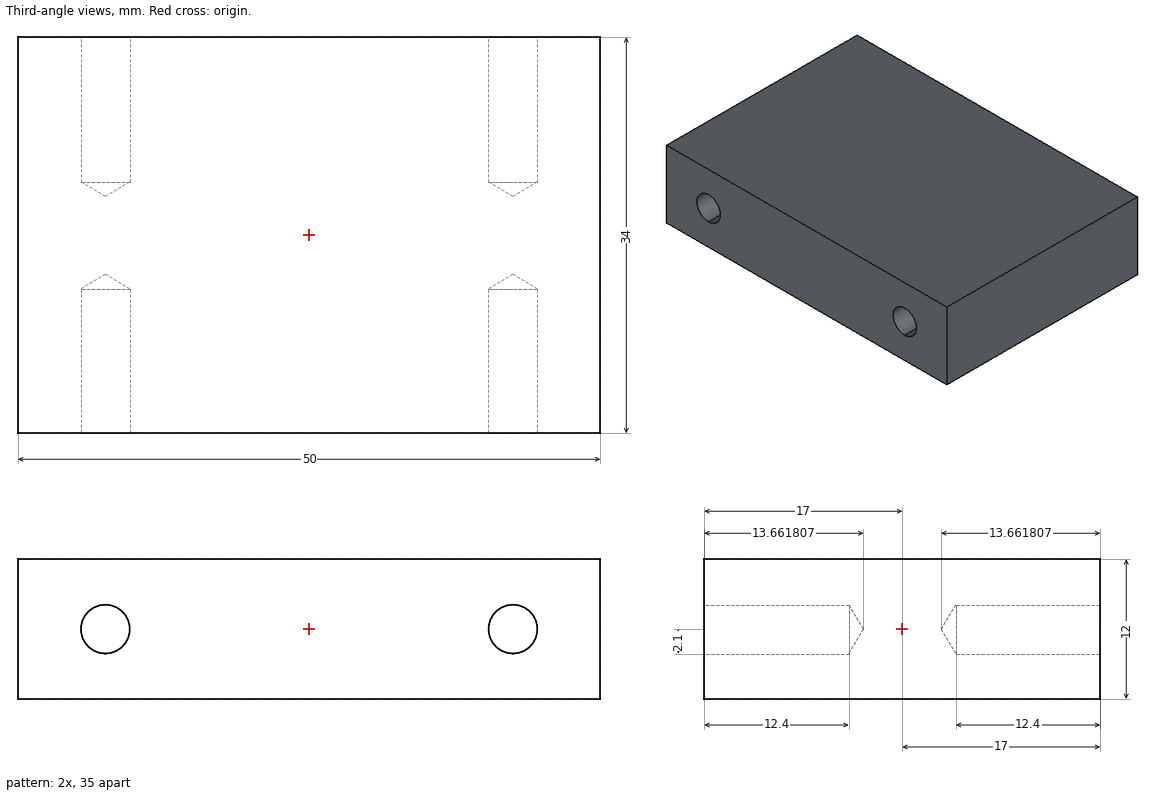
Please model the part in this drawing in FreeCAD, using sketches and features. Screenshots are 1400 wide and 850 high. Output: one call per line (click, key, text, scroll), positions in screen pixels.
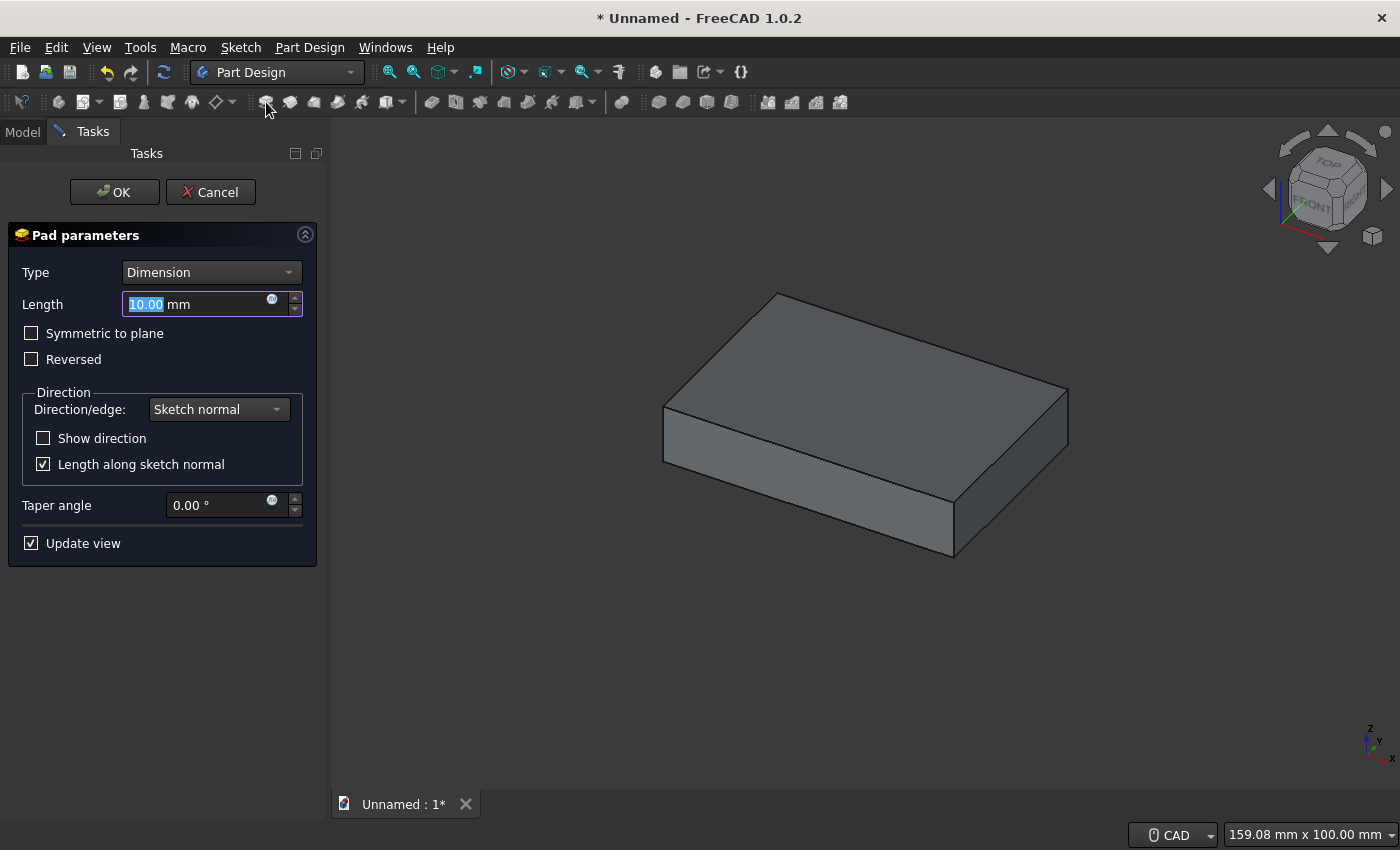
text(12)
key(Tab)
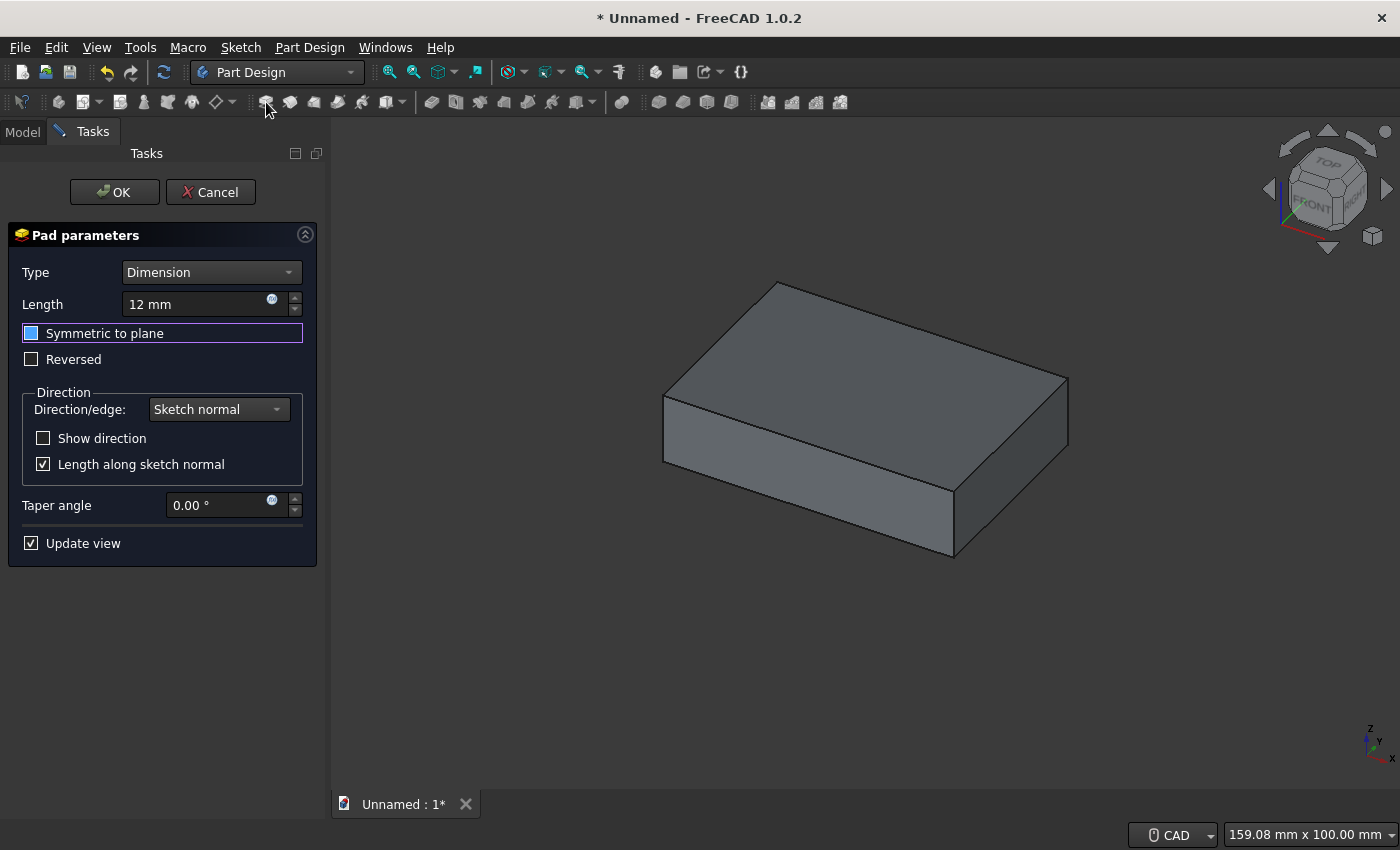
click(30, 333)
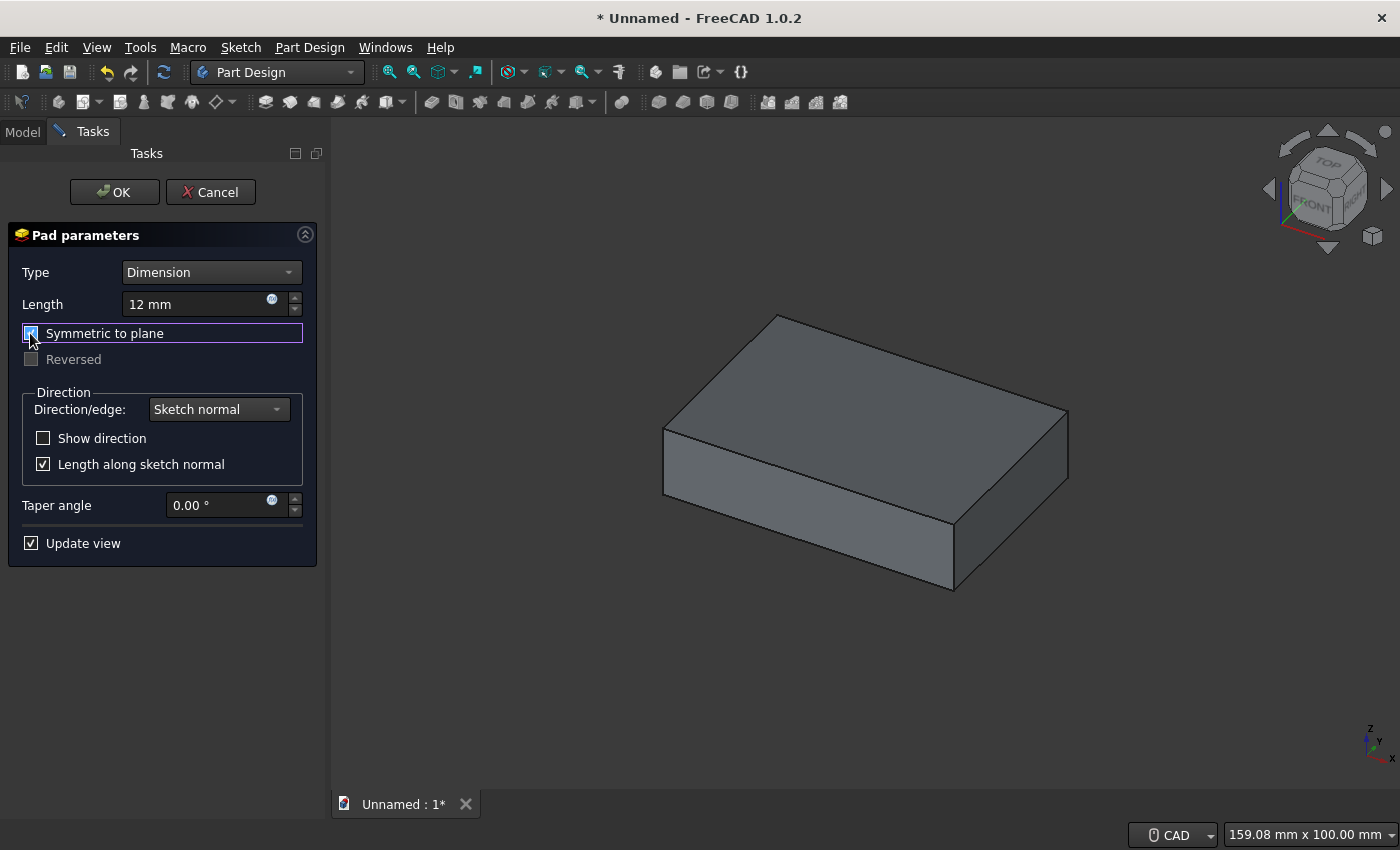
click(115, 192)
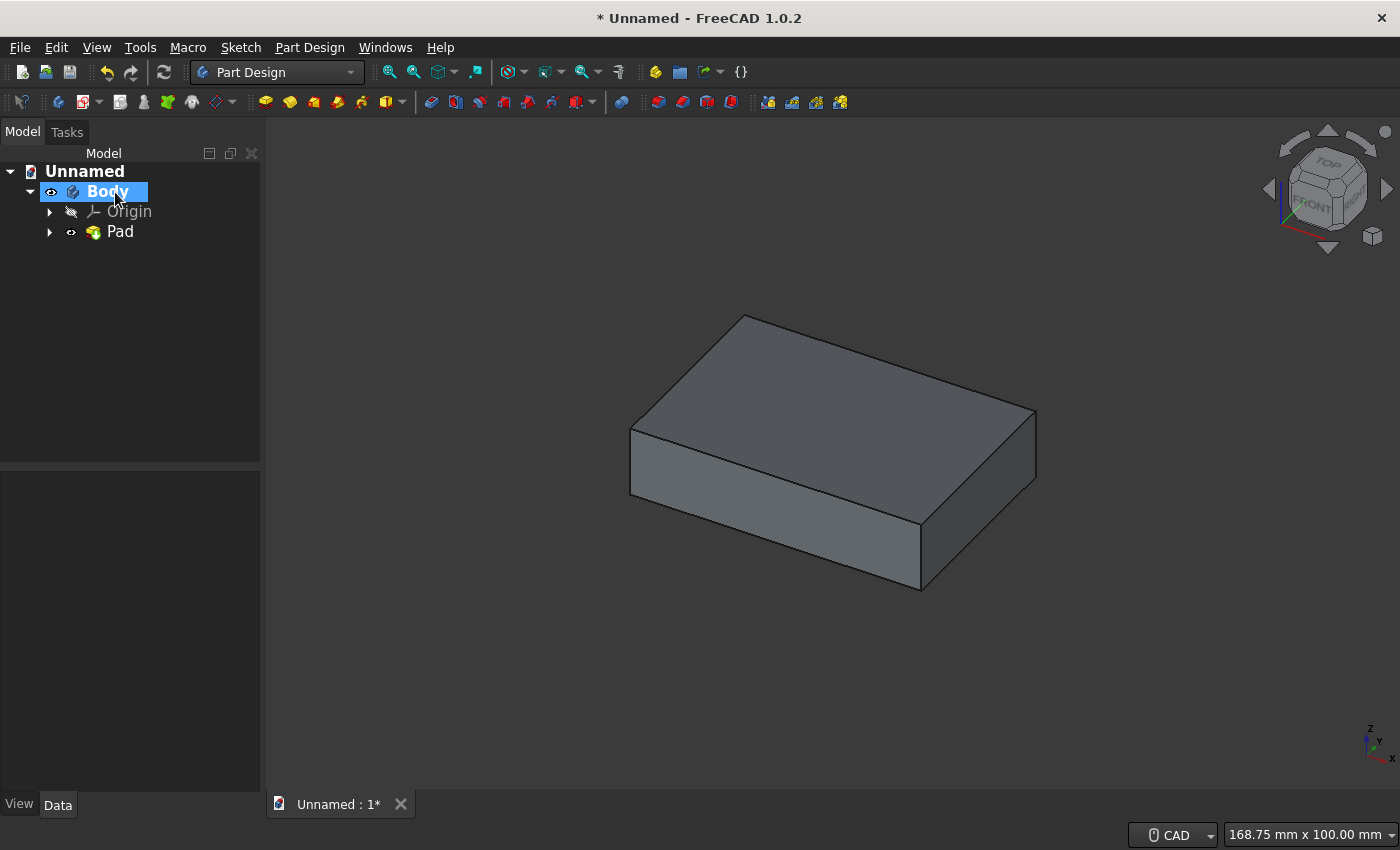
click(390, 72)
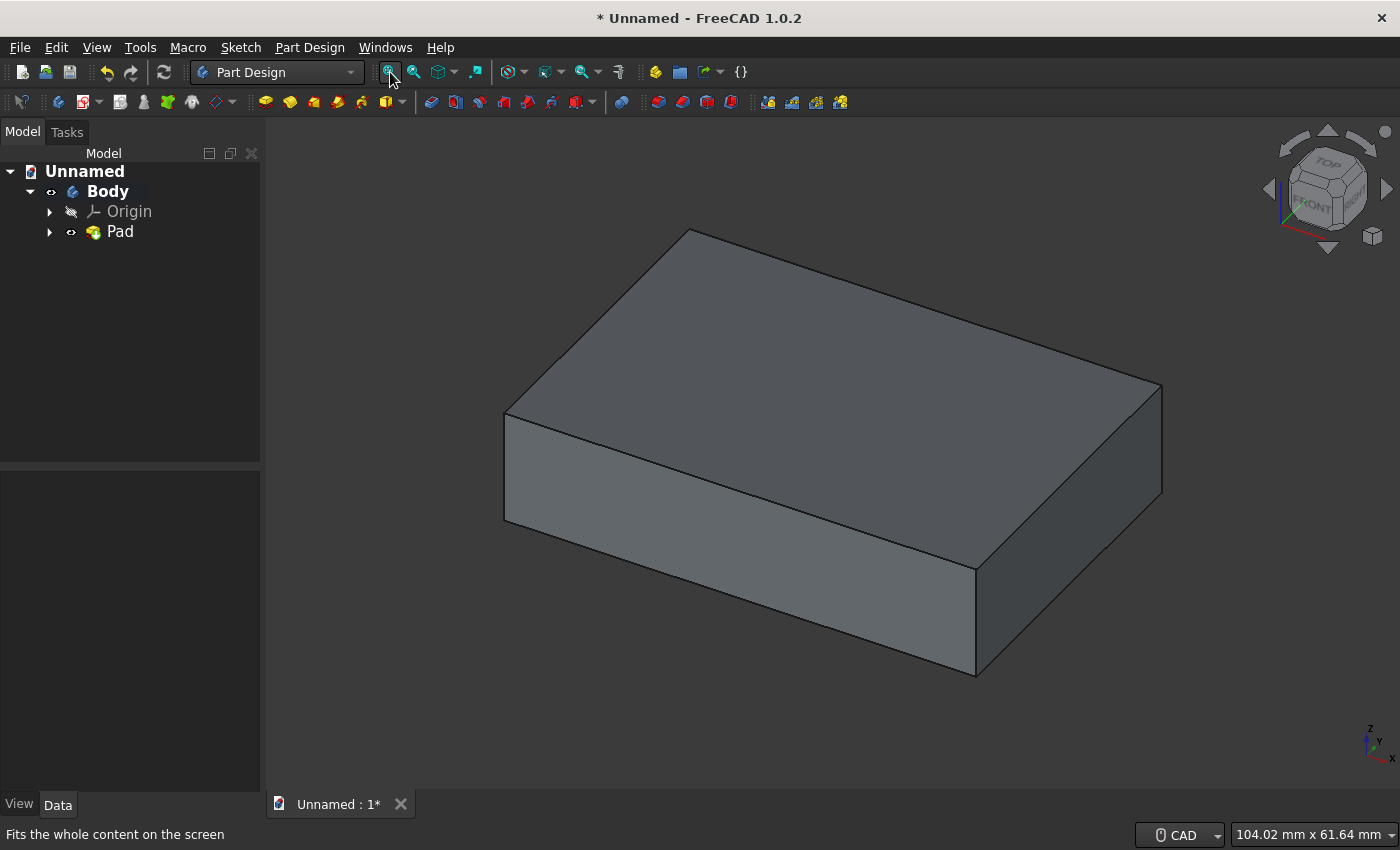
click(50, 212)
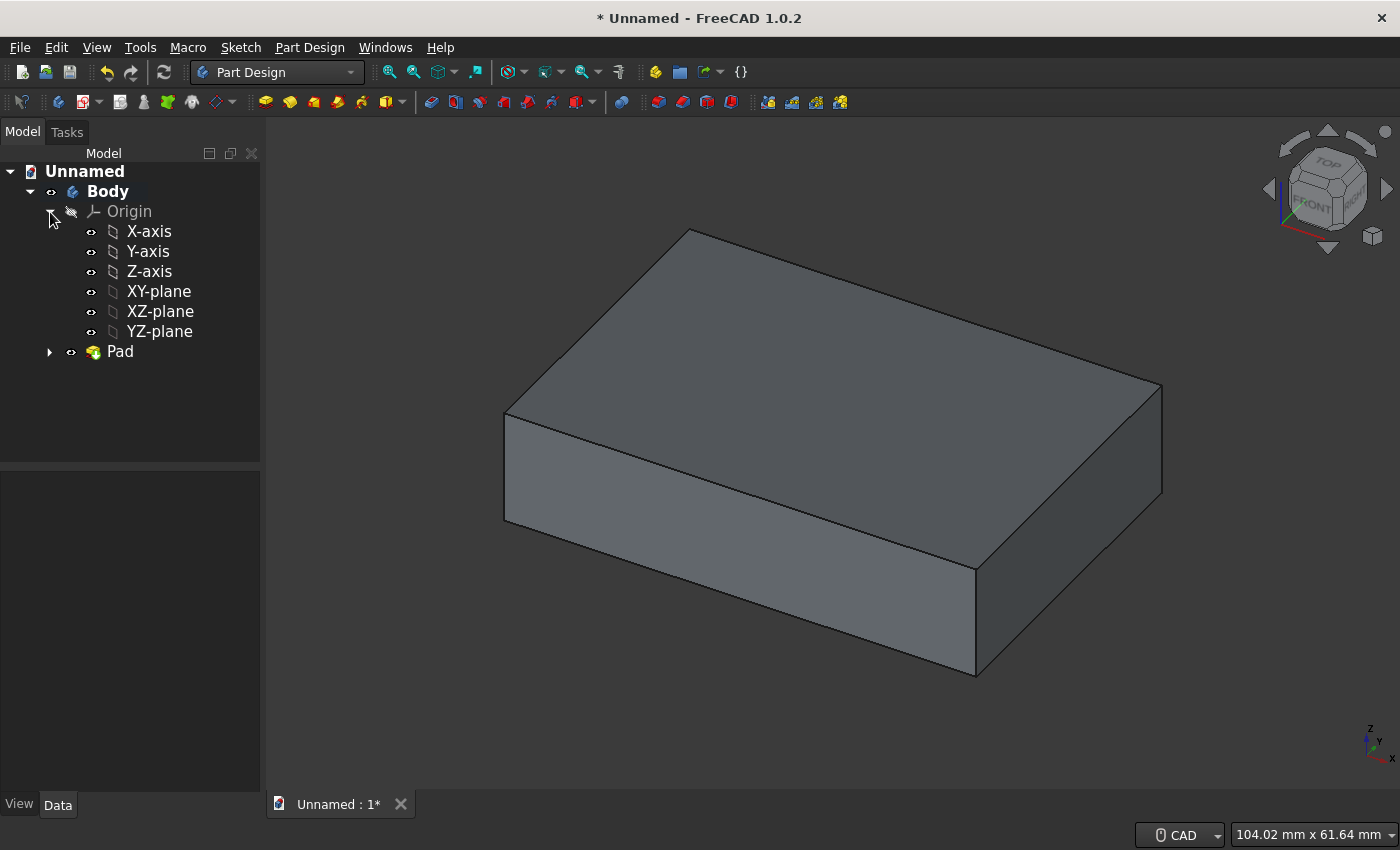
click(136, 332)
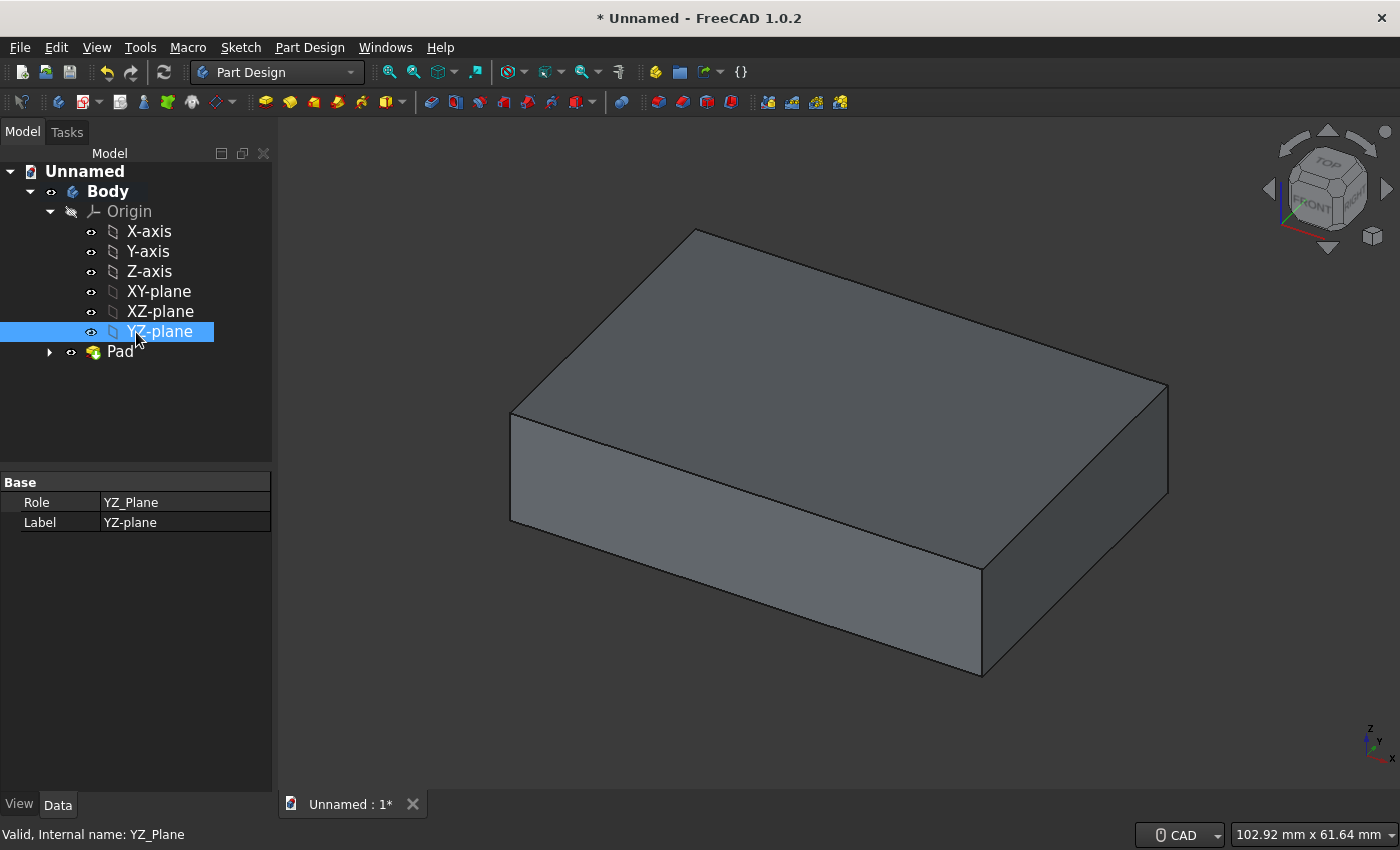
click(216, 102)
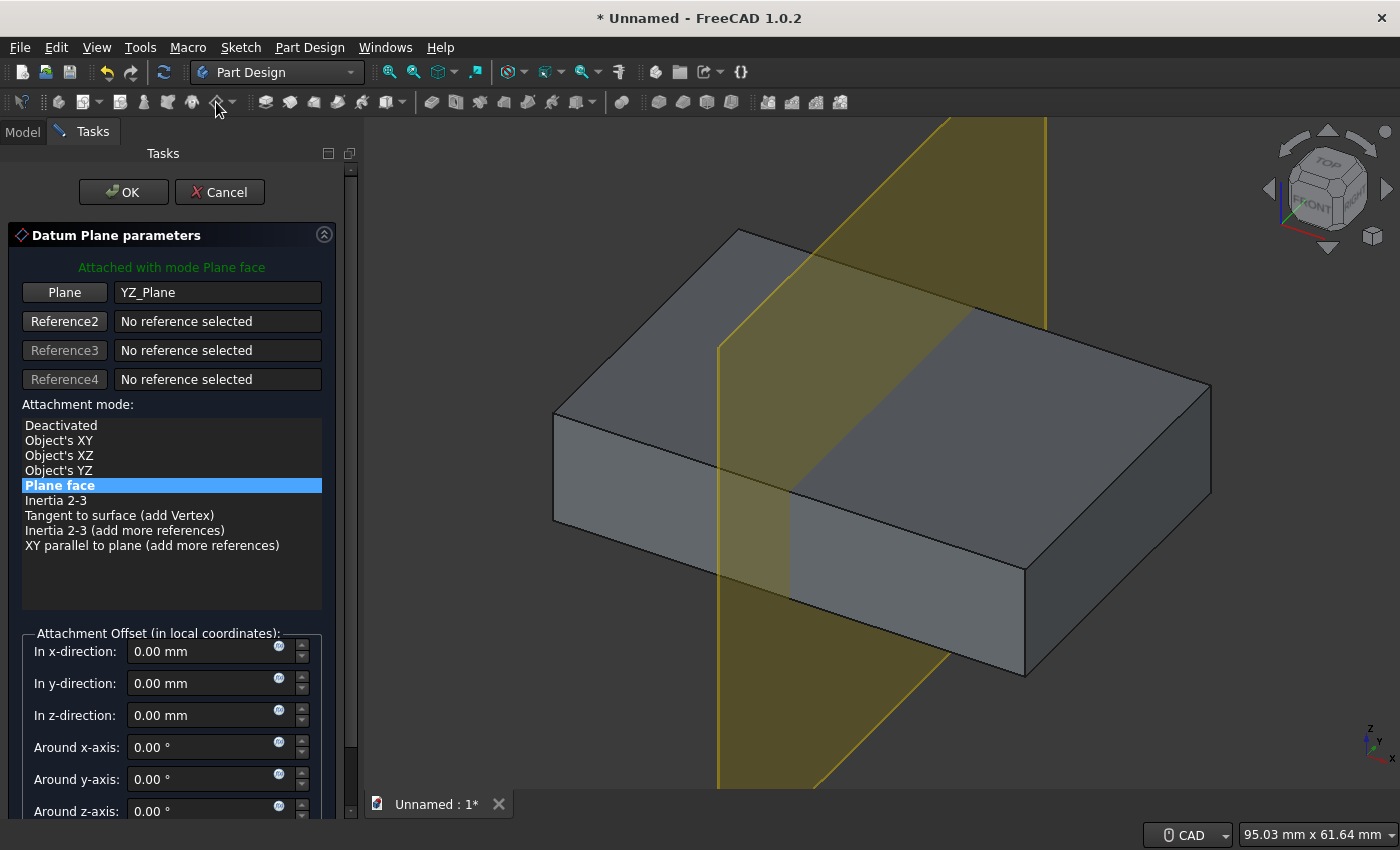
triple_click(210, 715)